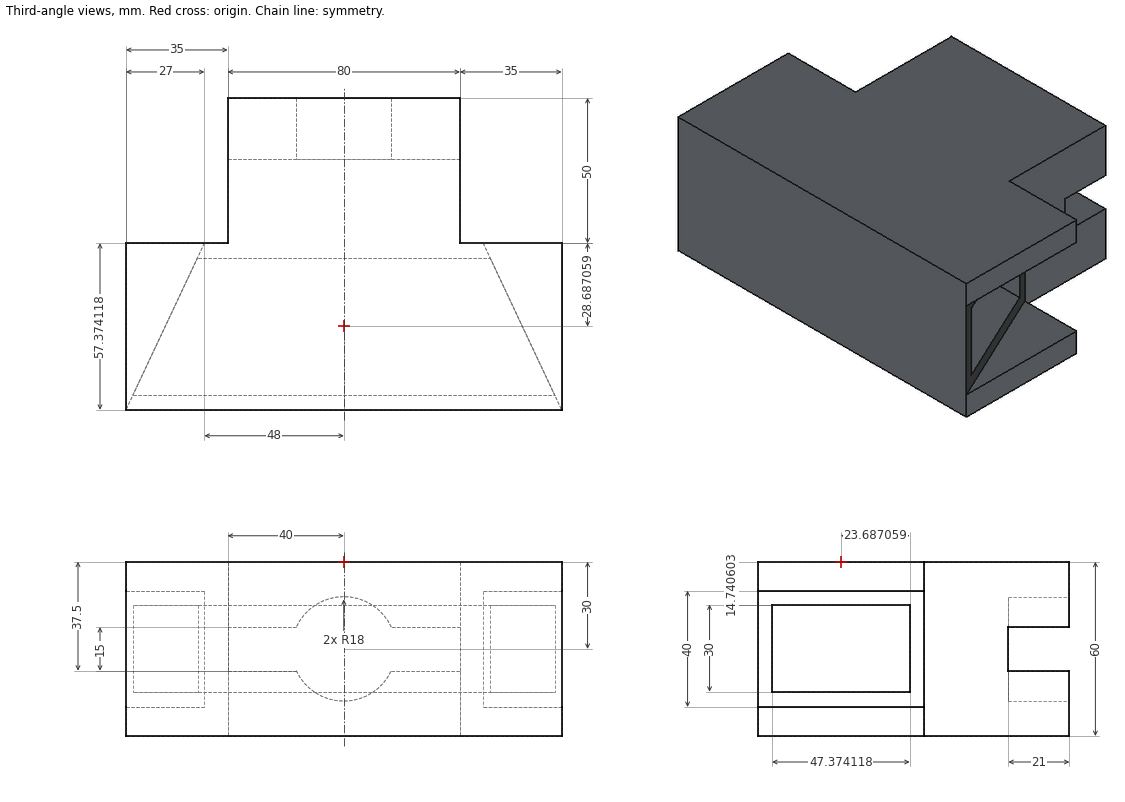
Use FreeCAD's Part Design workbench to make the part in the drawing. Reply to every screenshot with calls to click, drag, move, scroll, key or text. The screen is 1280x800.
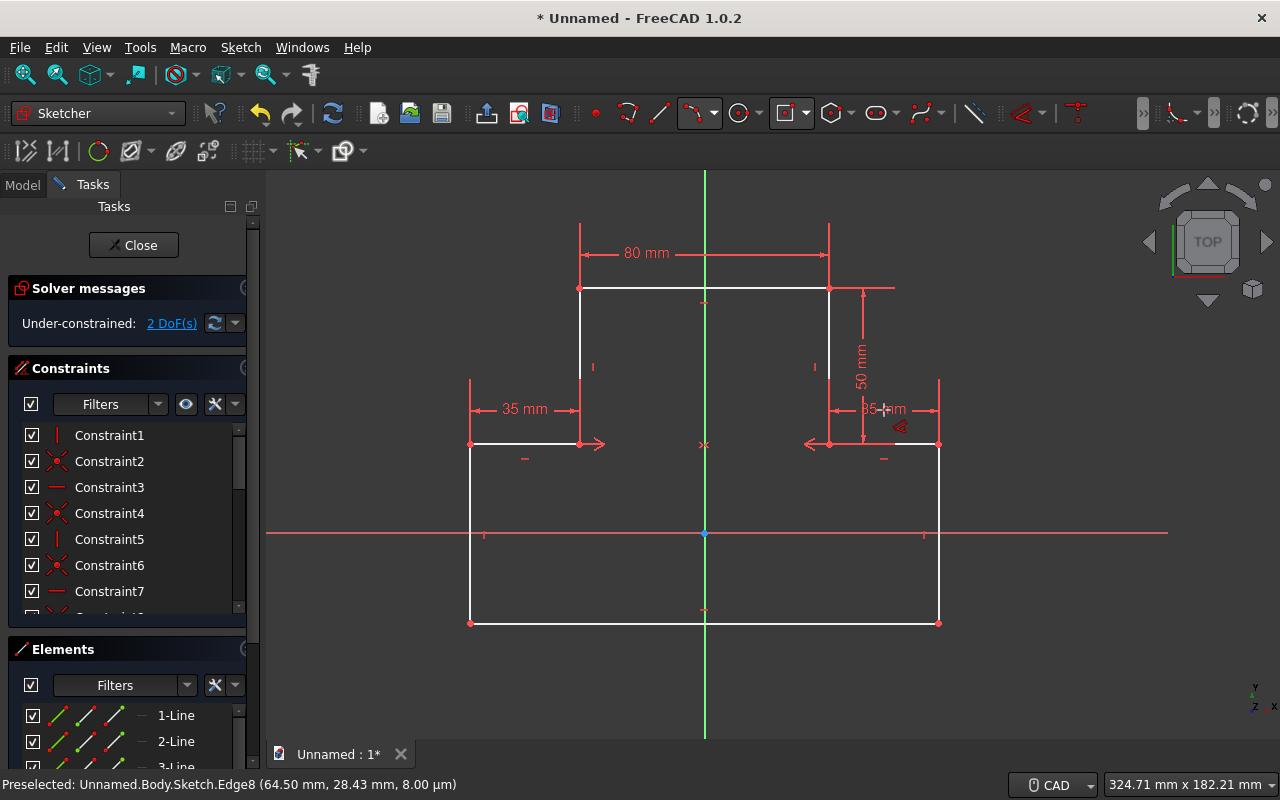
click(470, 498)
click(436, 493)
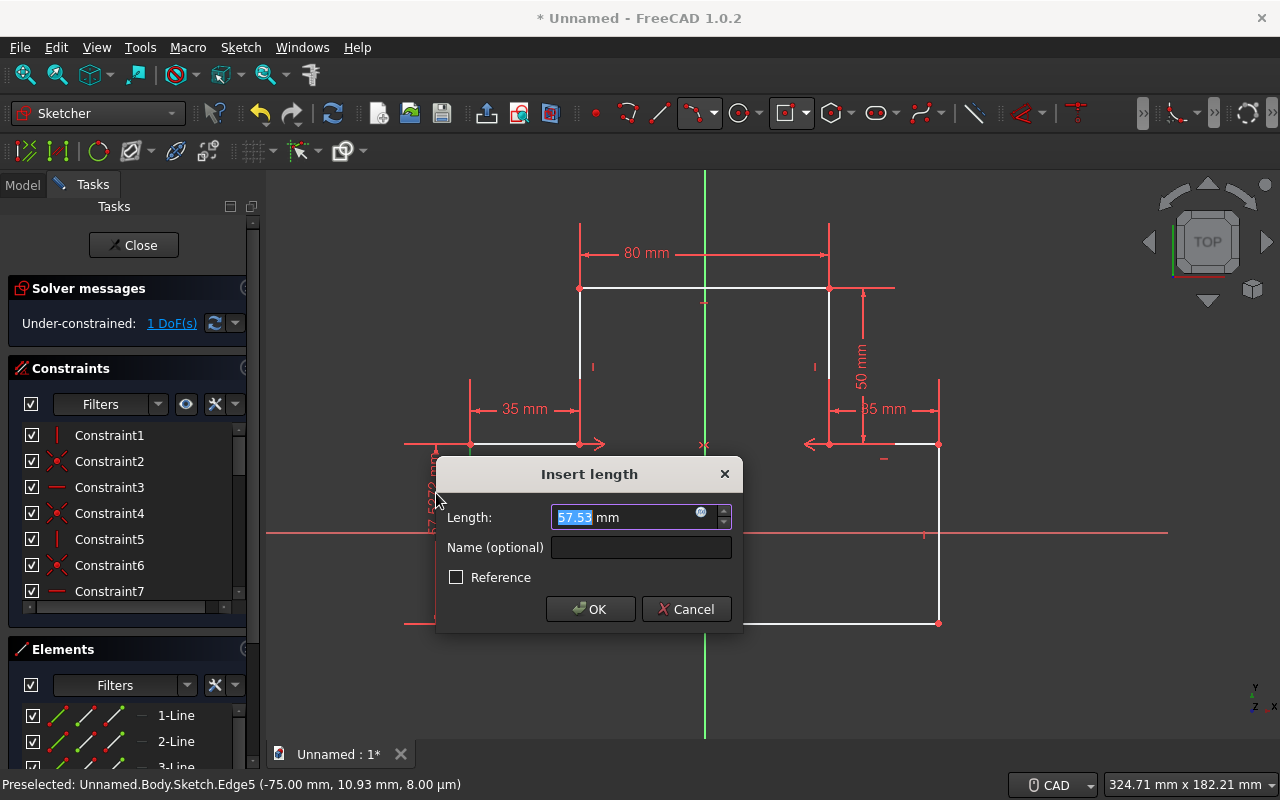
text(57.374118)
key(Return)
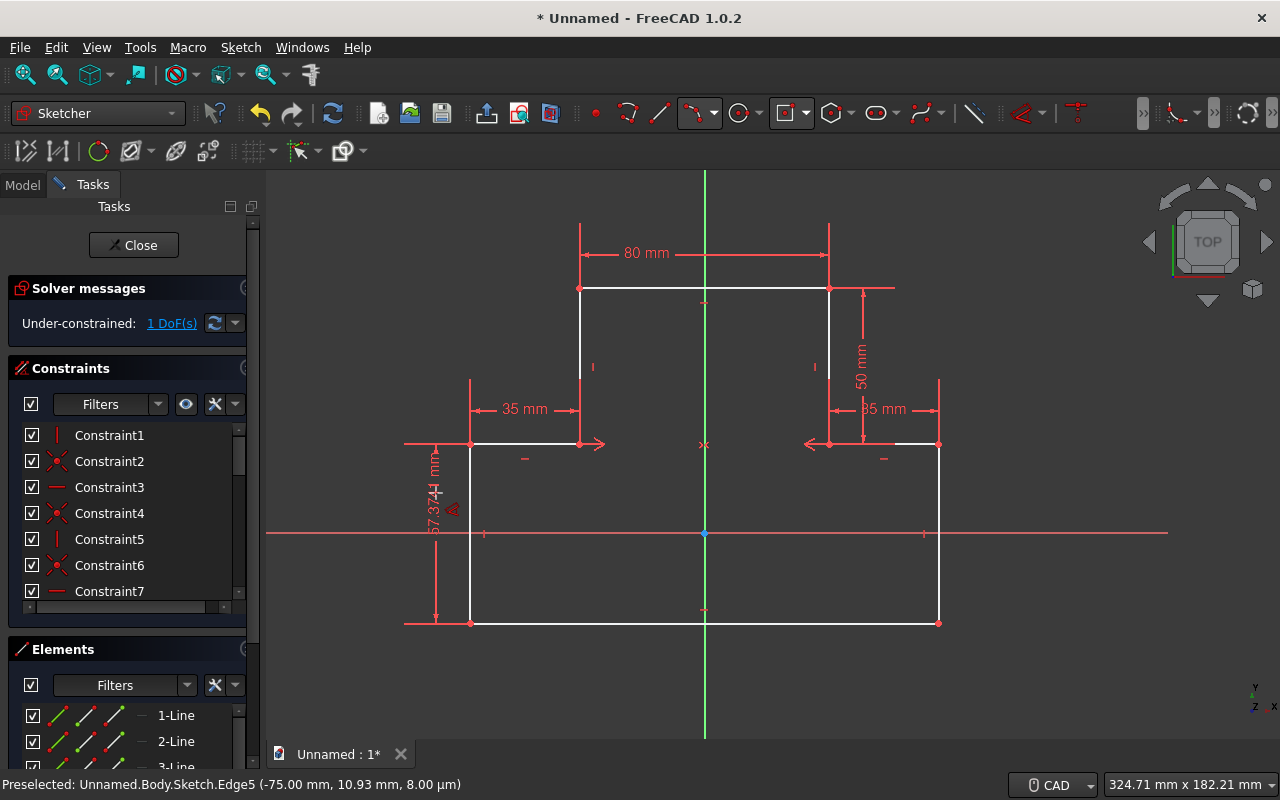
click(829, 444)
click(863, 489)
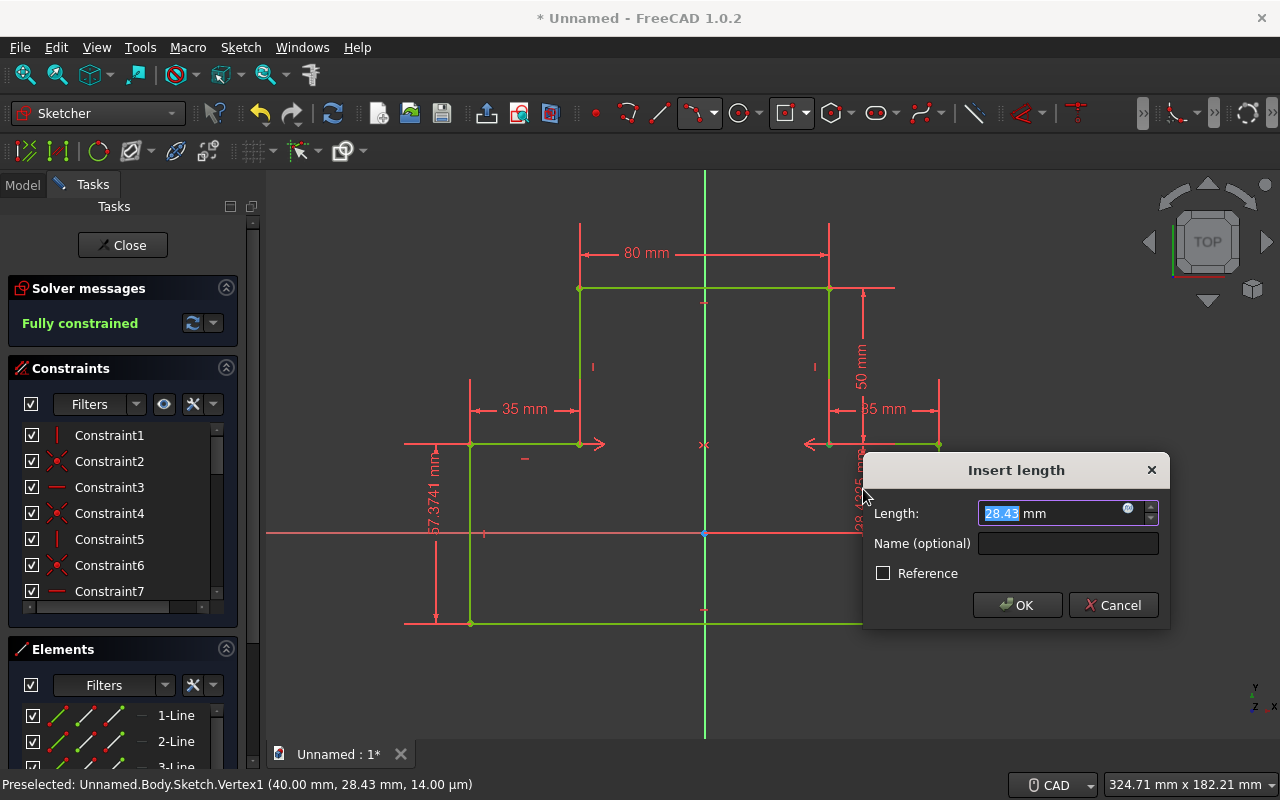
text(28.687059)
key(Return)
key(Escape)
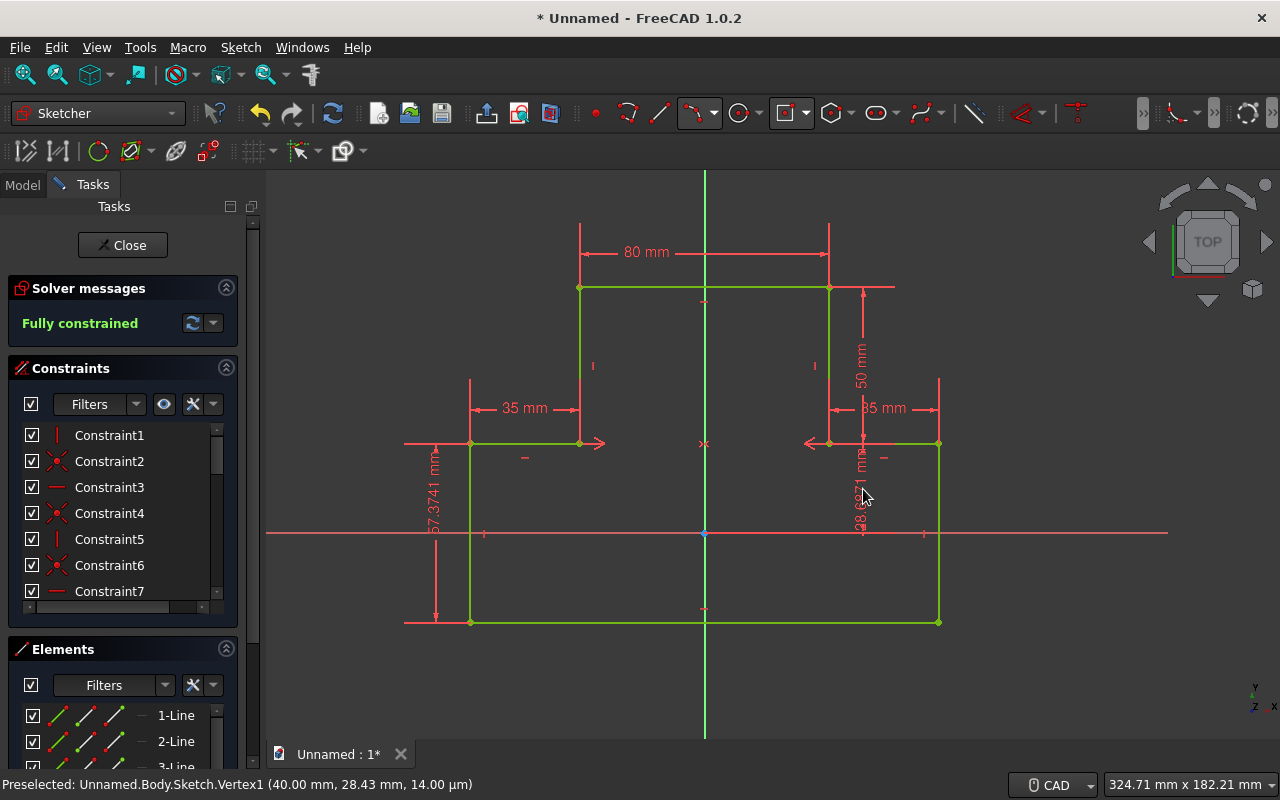
click(123, 245)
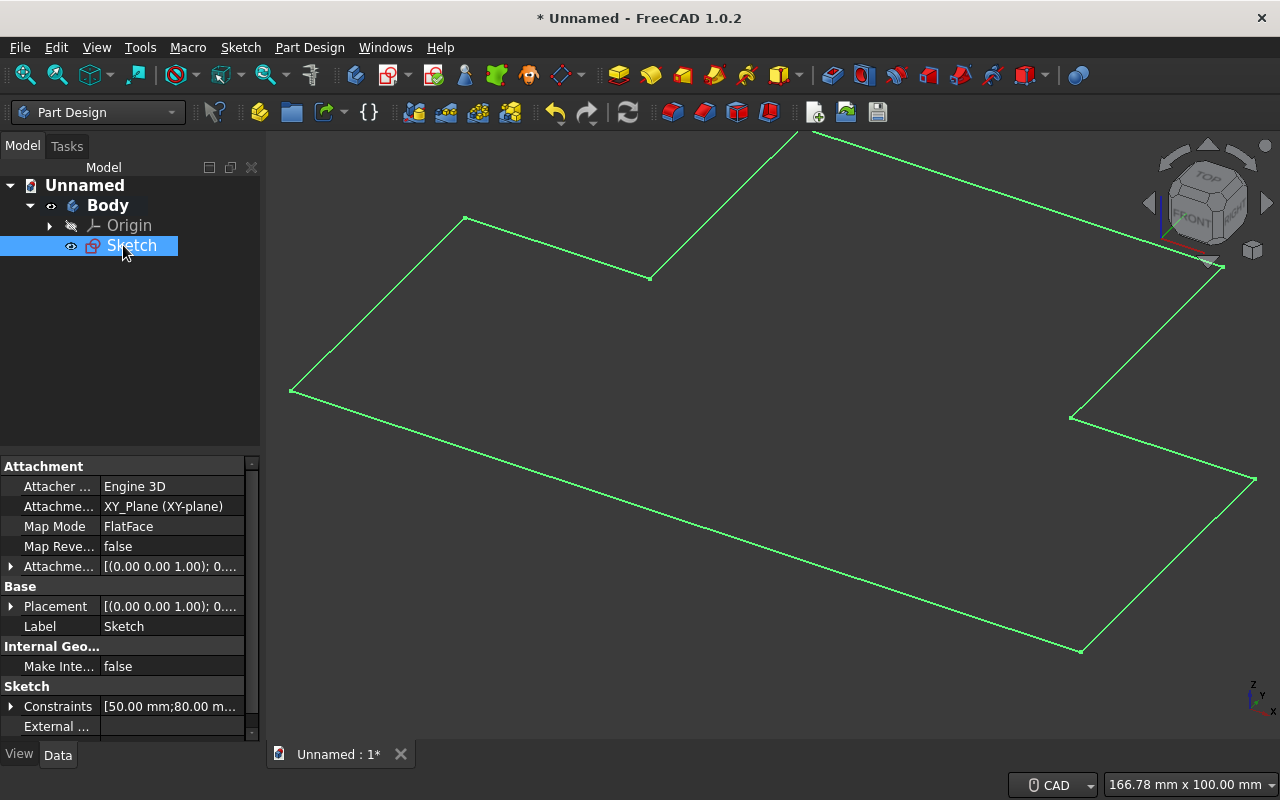
click(620, 76)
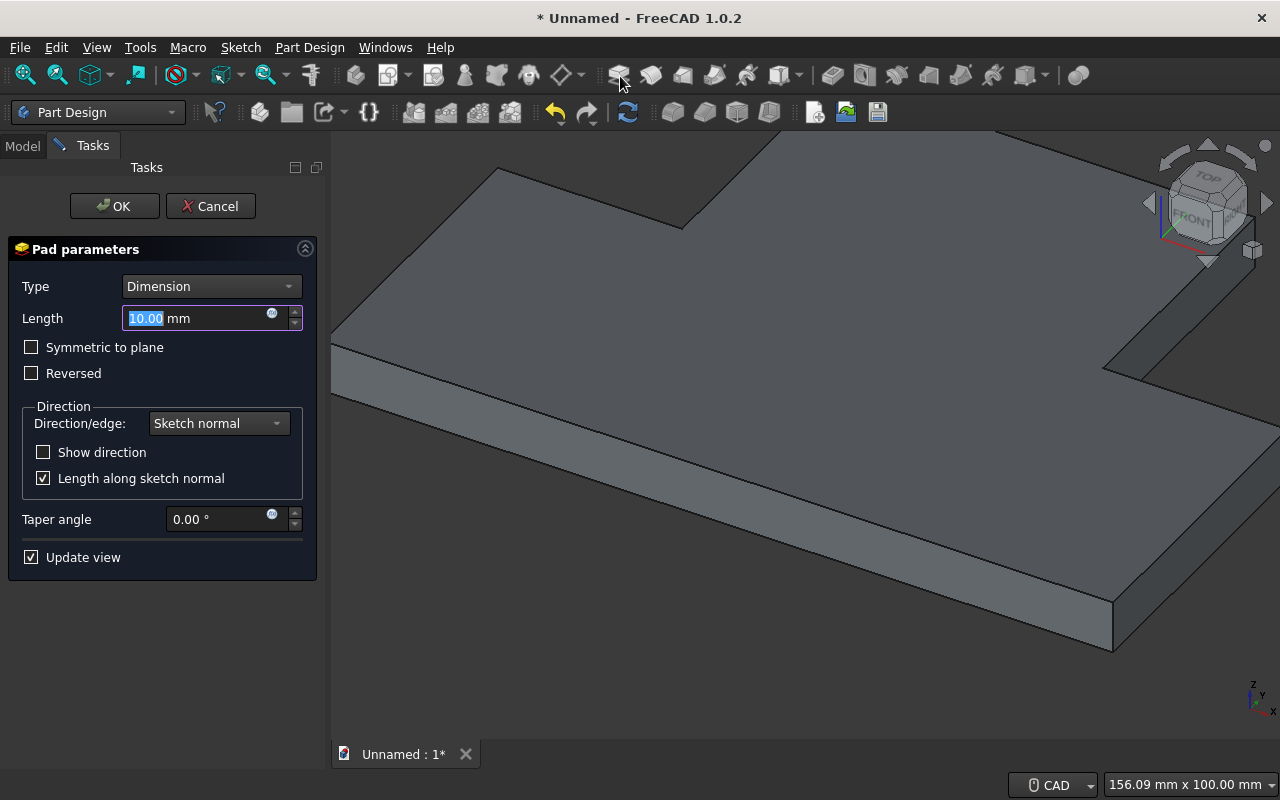
text(60)
key(Tab)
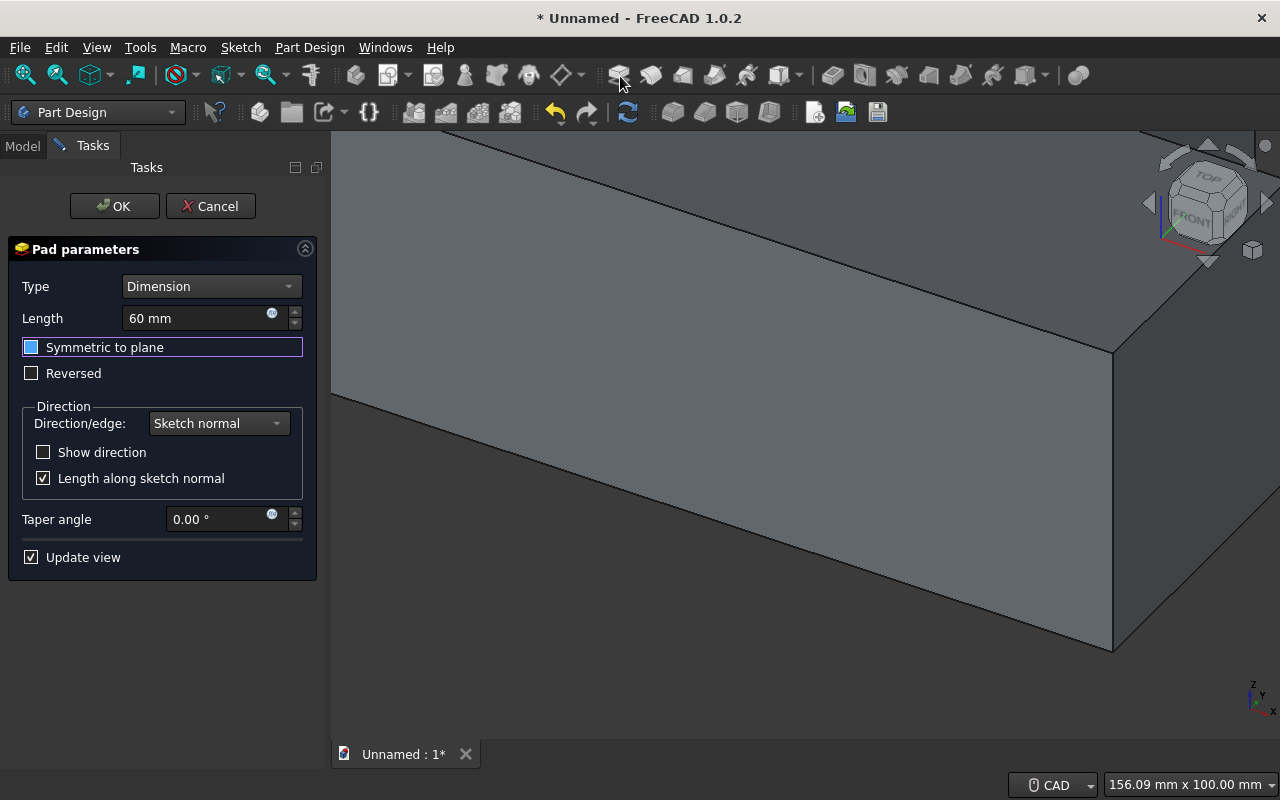
click(30, 373)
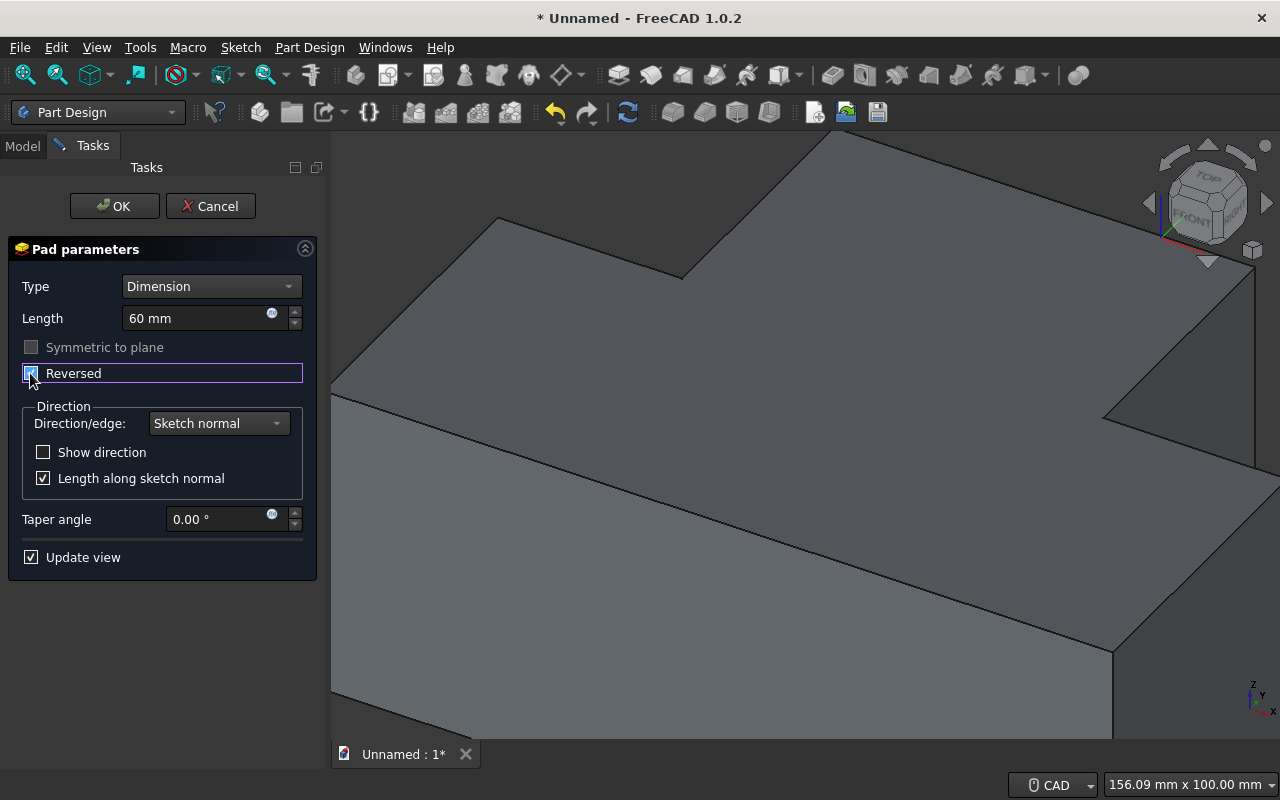
click(115, 206)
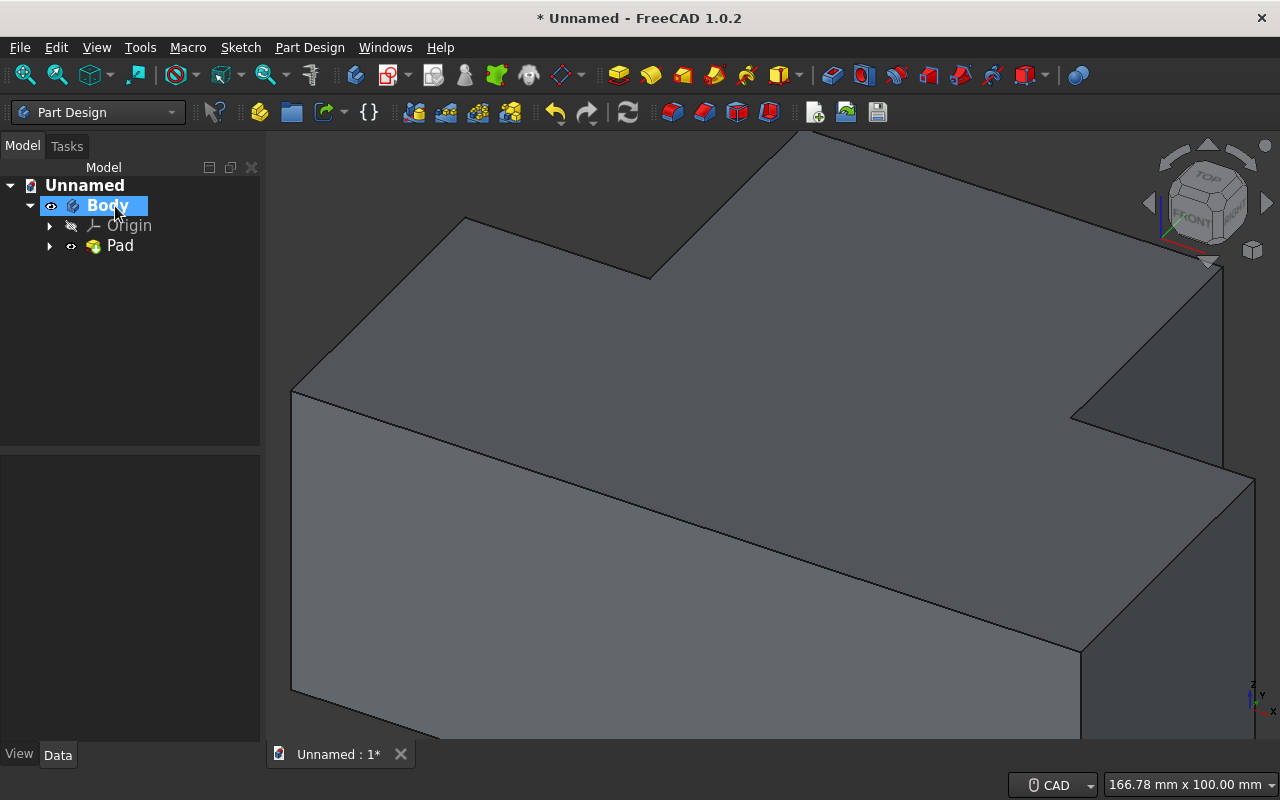
key(v)
key(f)